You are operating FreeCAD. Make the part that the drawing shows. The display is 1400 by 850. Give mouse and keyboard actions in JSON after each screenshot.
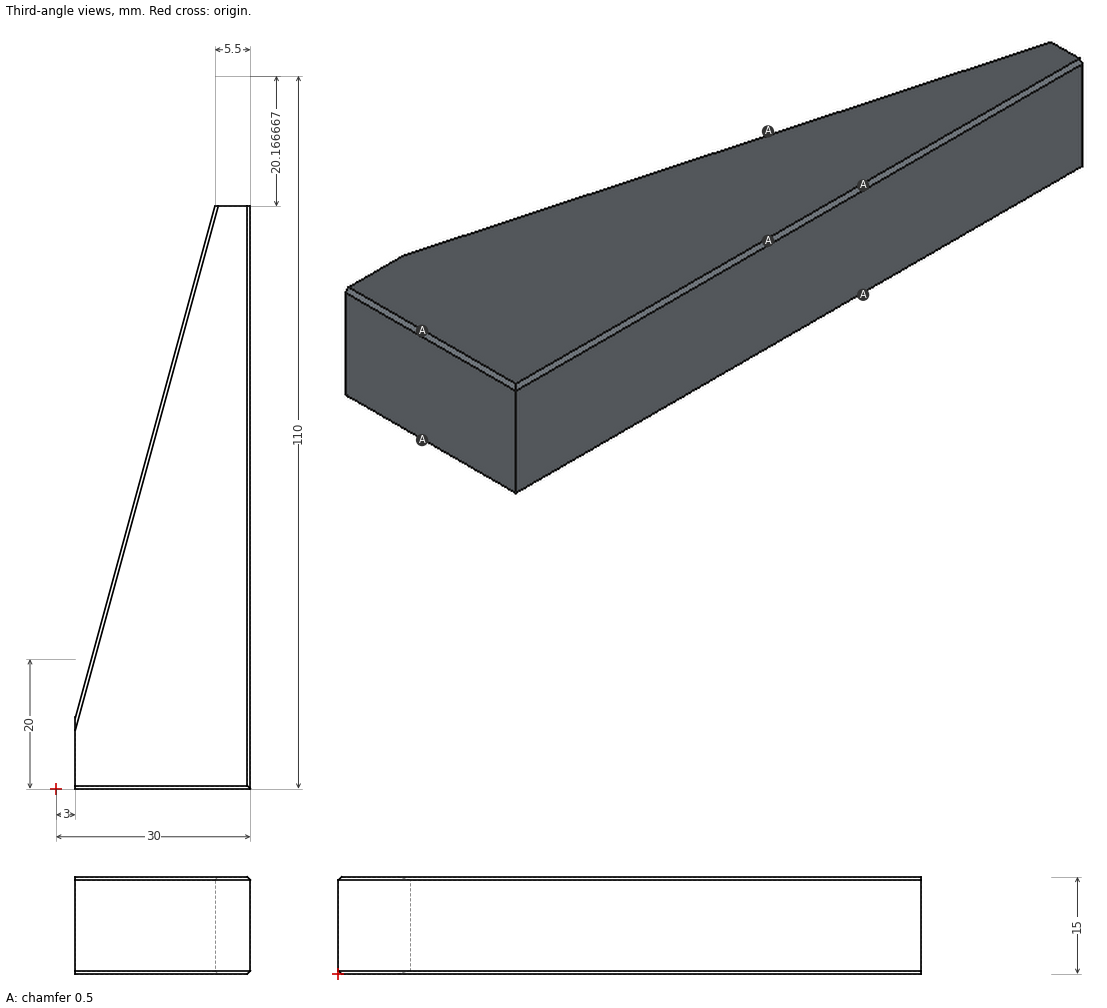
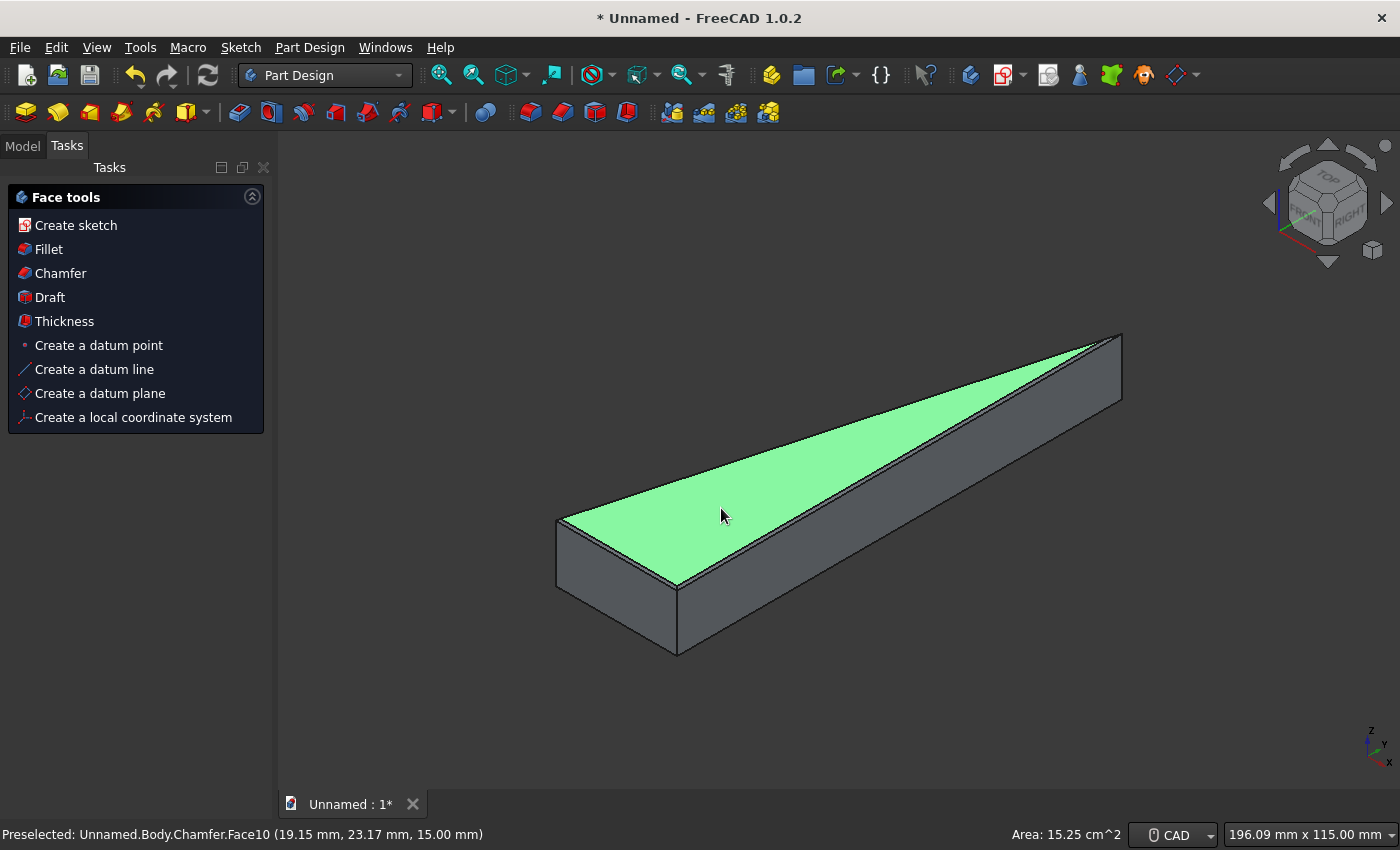
{"action": "left_click", "coordinate": [1004, 76]}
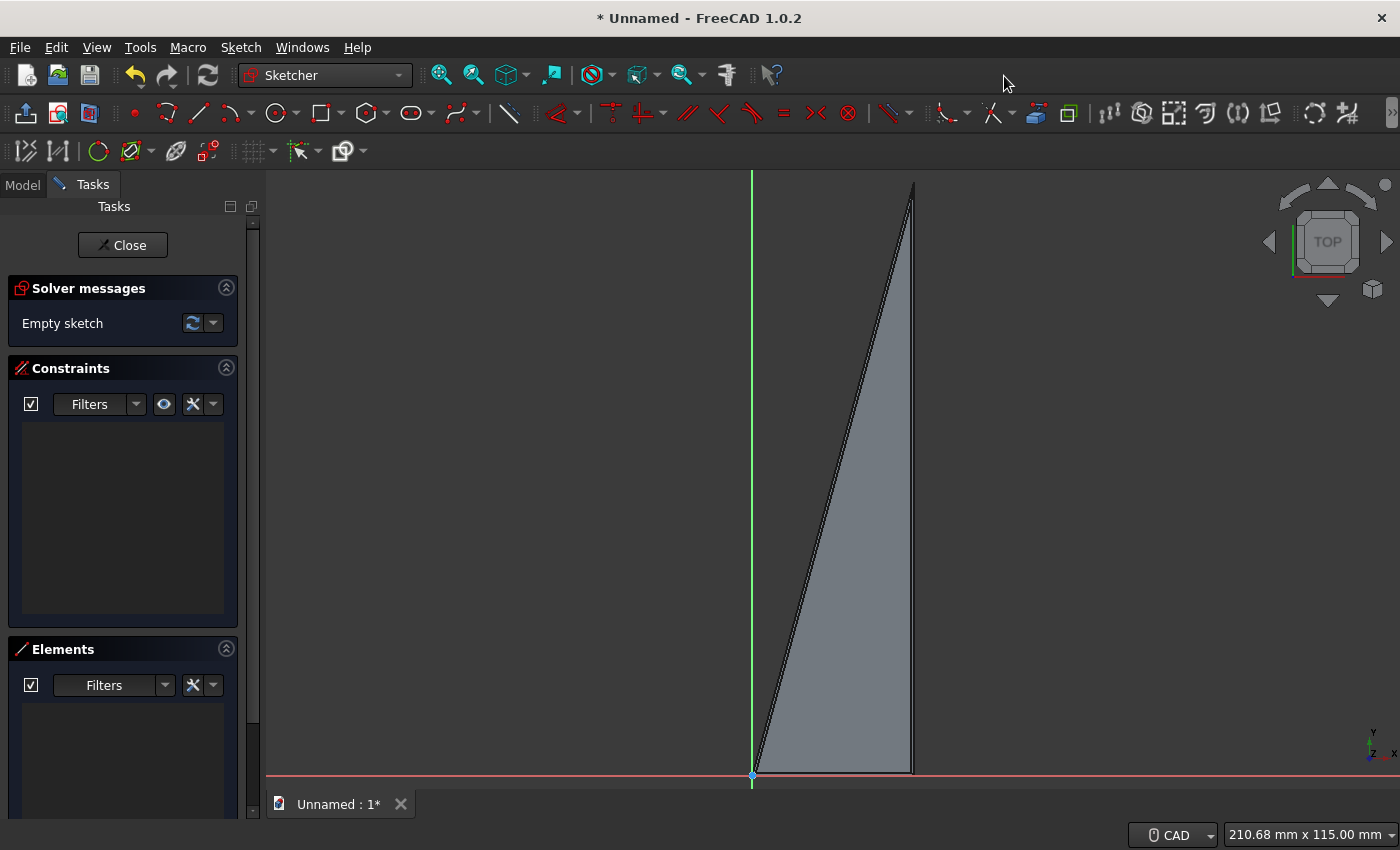
{"action": "scroll", "coordinate": [625, 480], "scroll_direction": "down", "scroll_amount": 2}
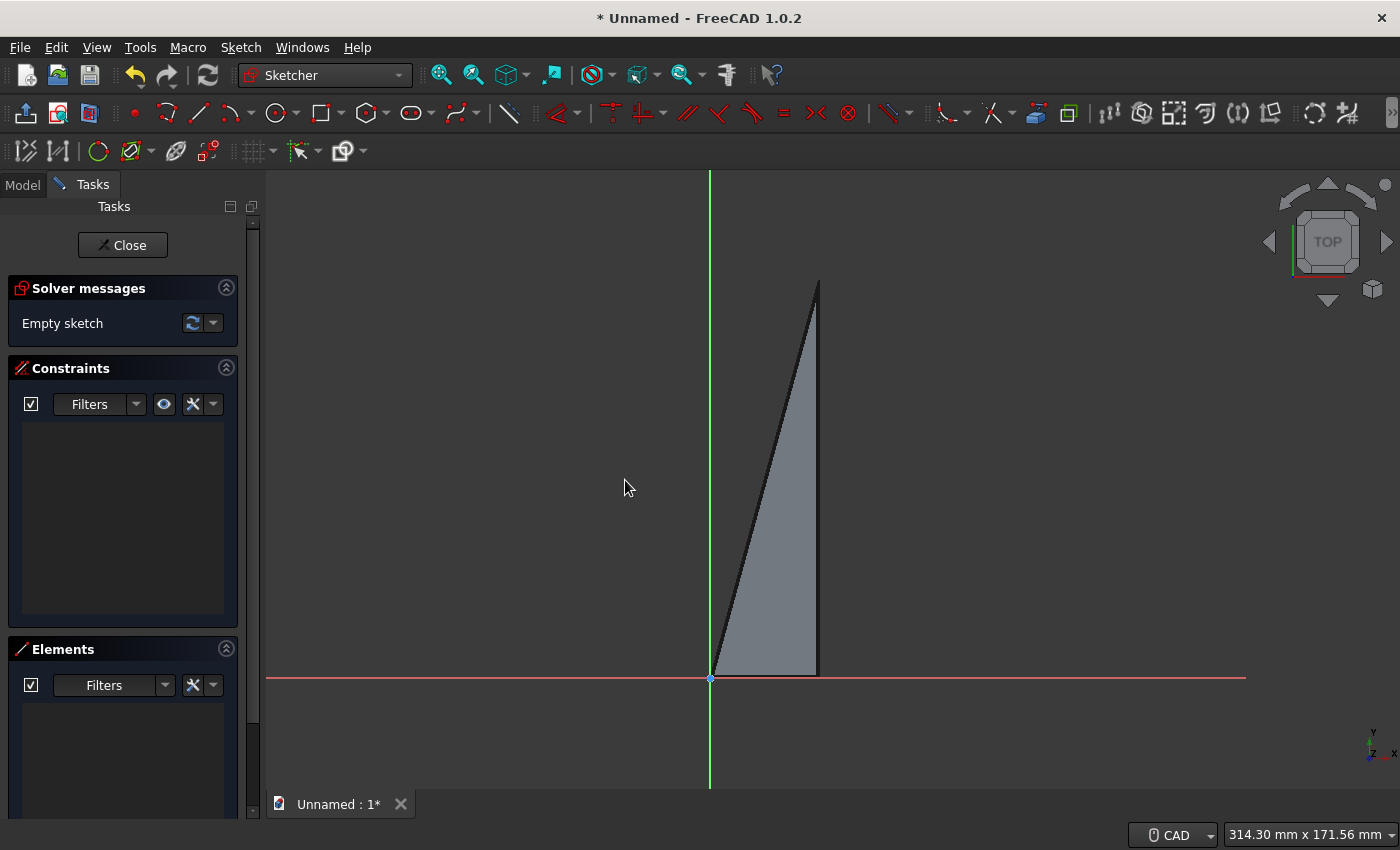
{"action": "left_click", "coordinate": [322, 114]}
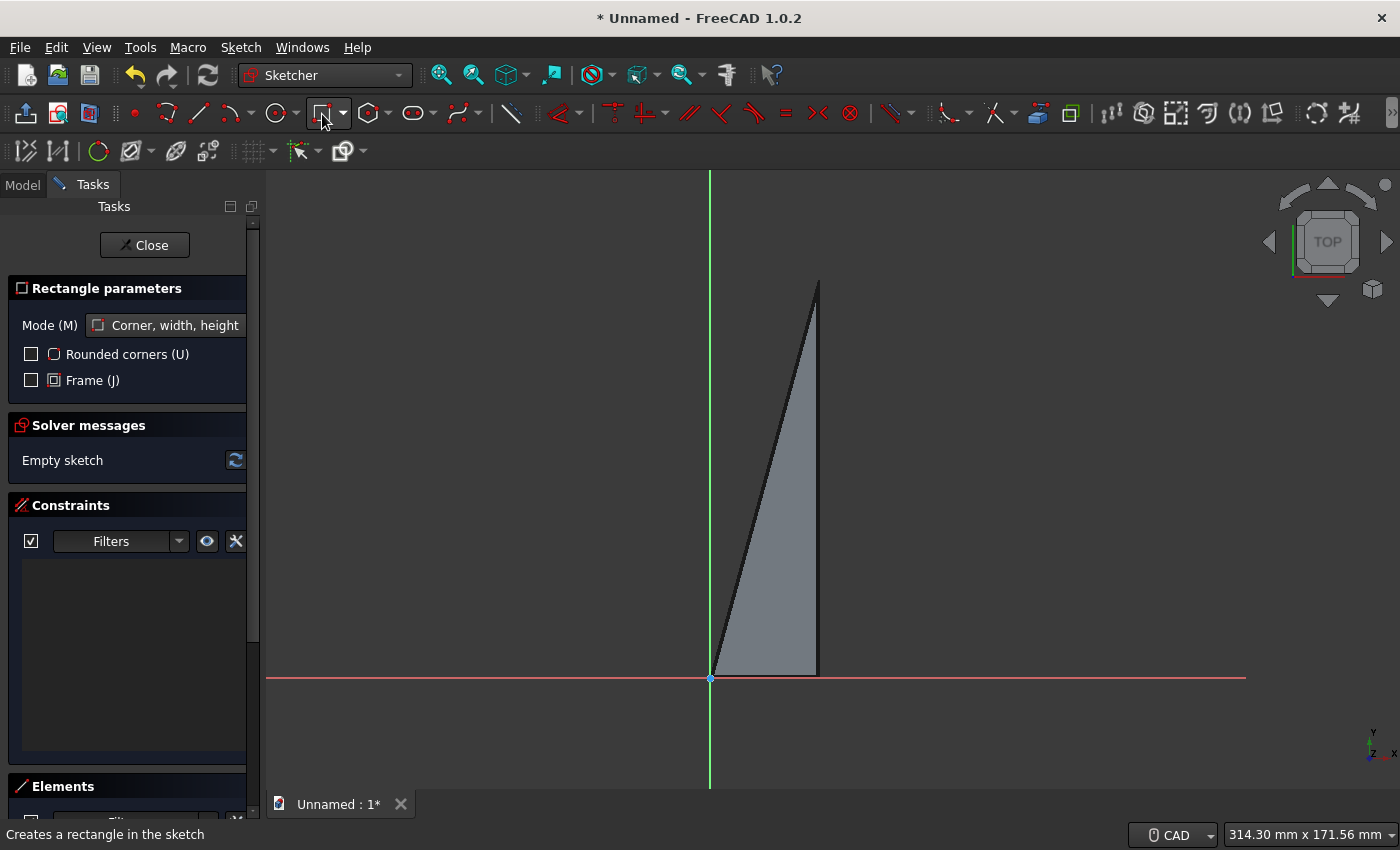
{"action": "left_click", "coordinate": [799, 281]}
{"action": "left_click", "coordinate": [819, 354]}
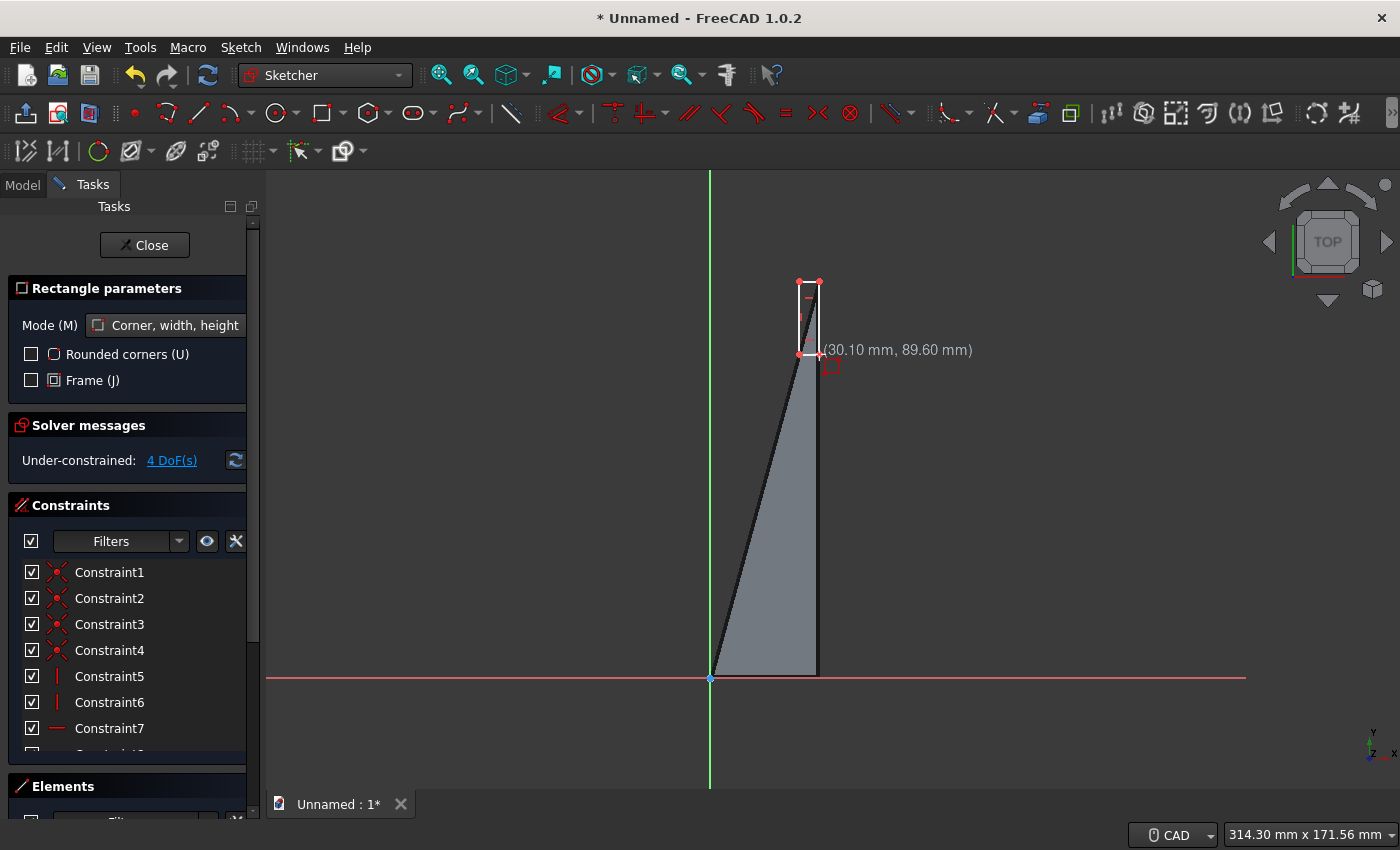
{"action": "scroll", "coordinate": [710, 678], "scroll_direction": "up", "scroll_amount": 2}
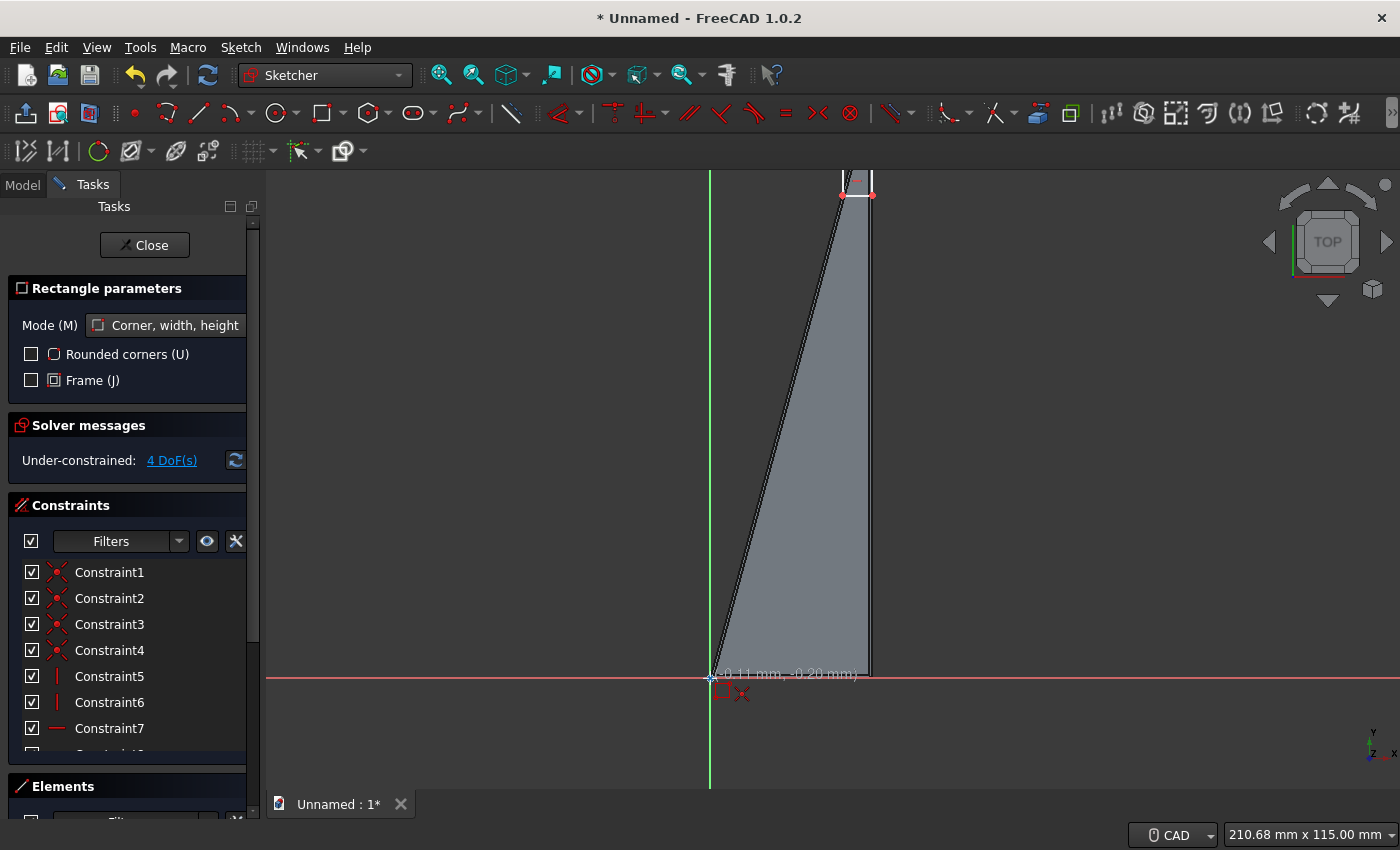
{"action": "left_click", "coordinate": [710, 678]}
{"action": "left_click", "coordinate": [727, 570]}
{"action": "key", "text": "Escape"}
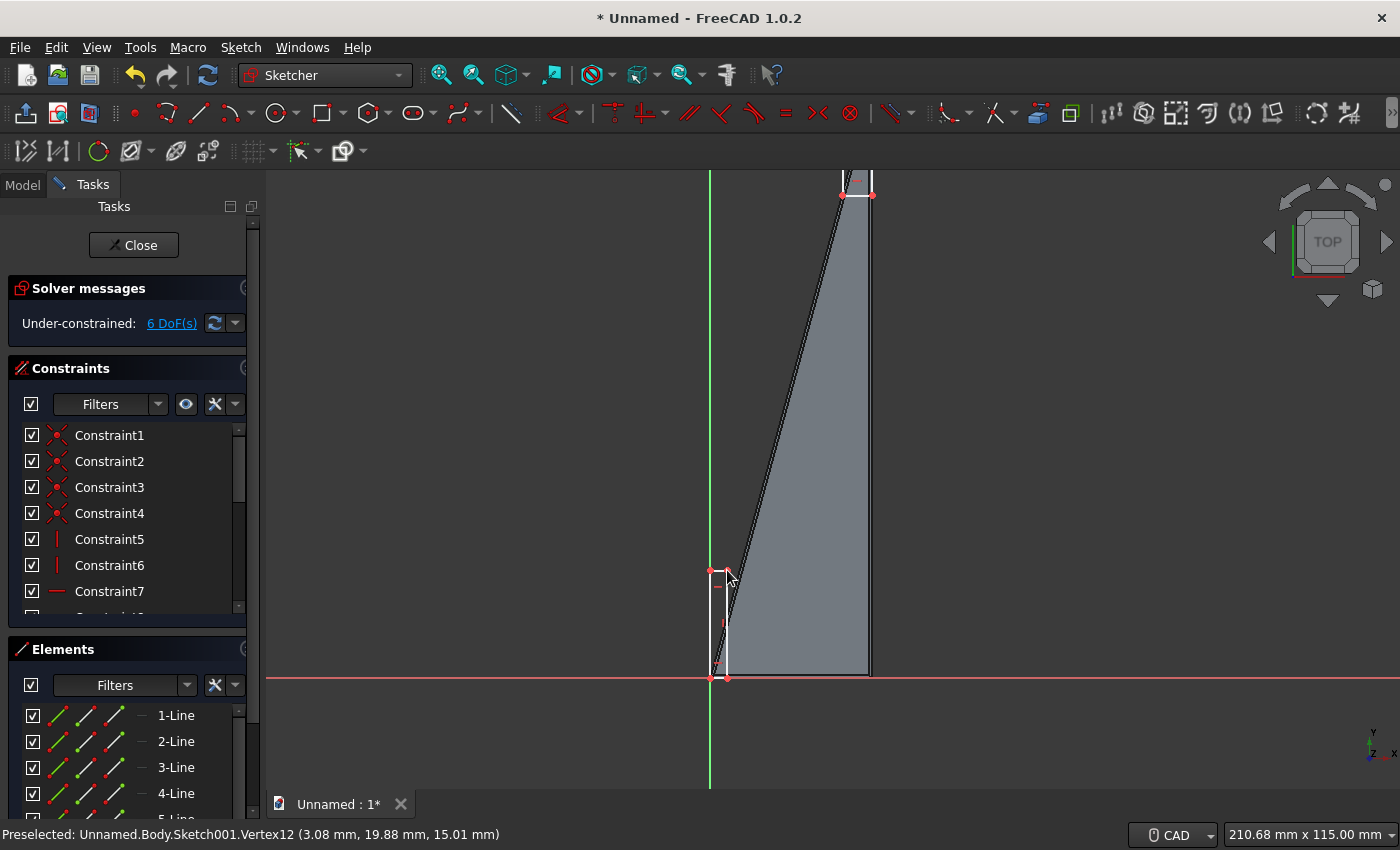
{"action": "left_click", "coordinate": [558, 114]}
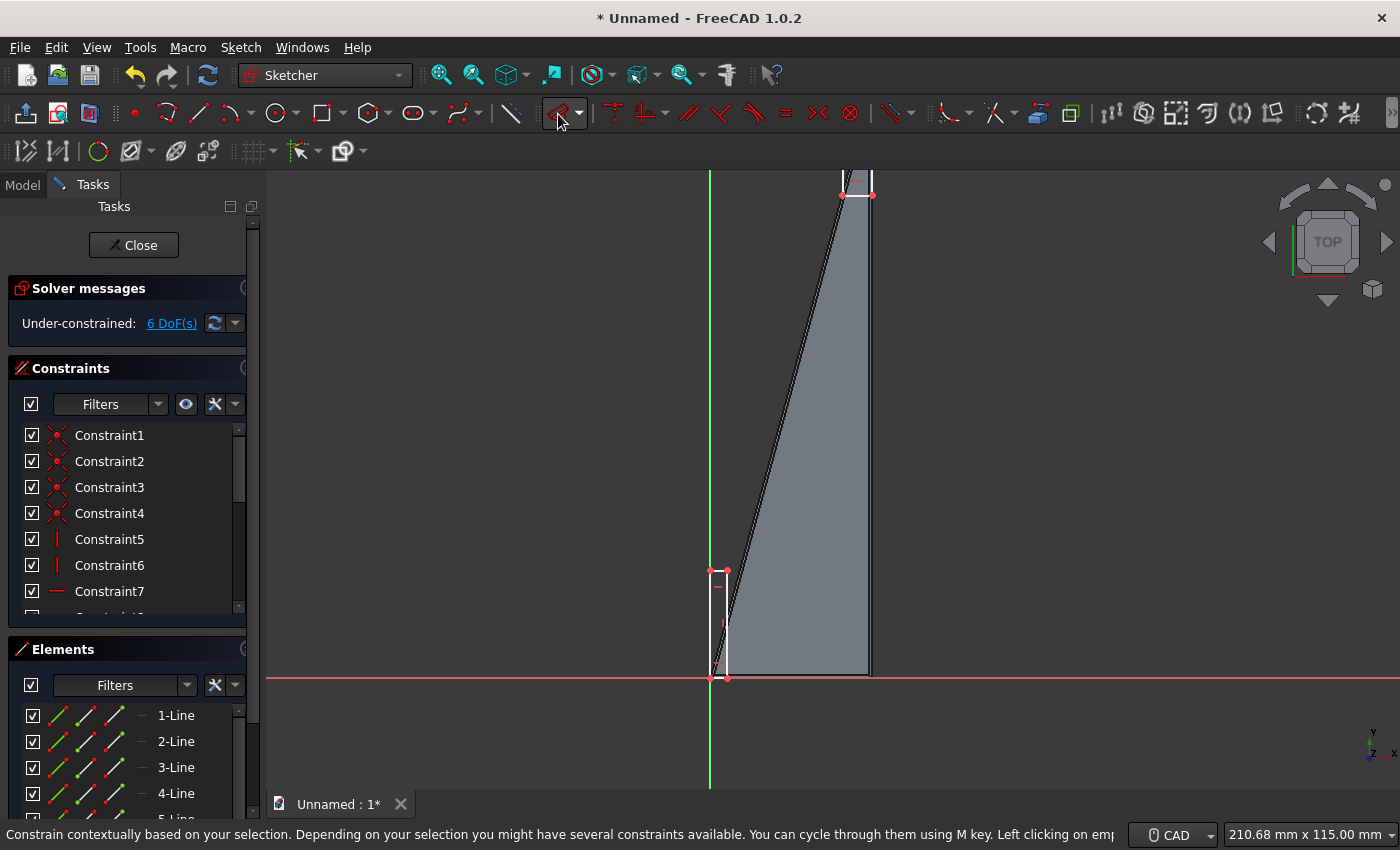
{"action": "scroll", "coordinate": [719, 678], "scroll_direction": "up", "scroll_amount": 5}